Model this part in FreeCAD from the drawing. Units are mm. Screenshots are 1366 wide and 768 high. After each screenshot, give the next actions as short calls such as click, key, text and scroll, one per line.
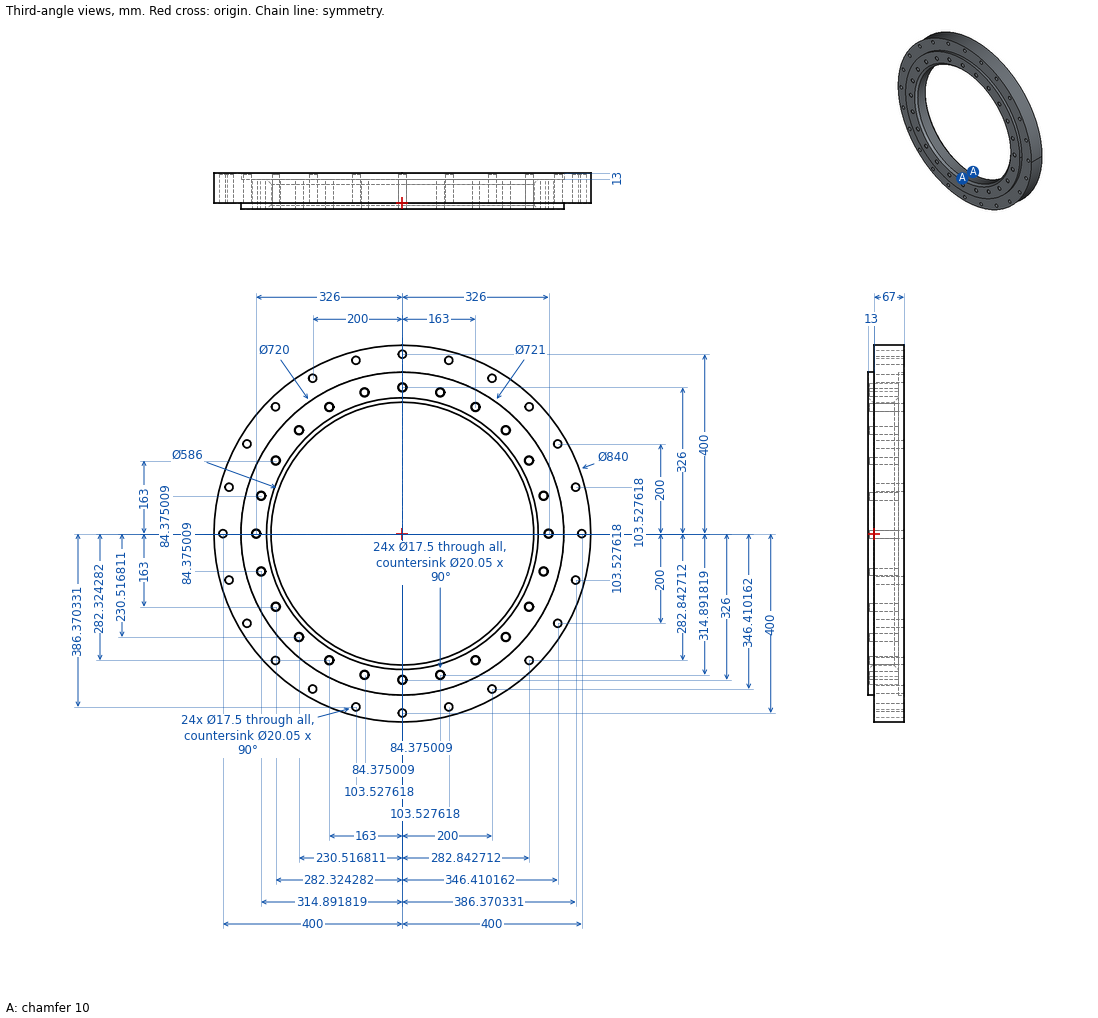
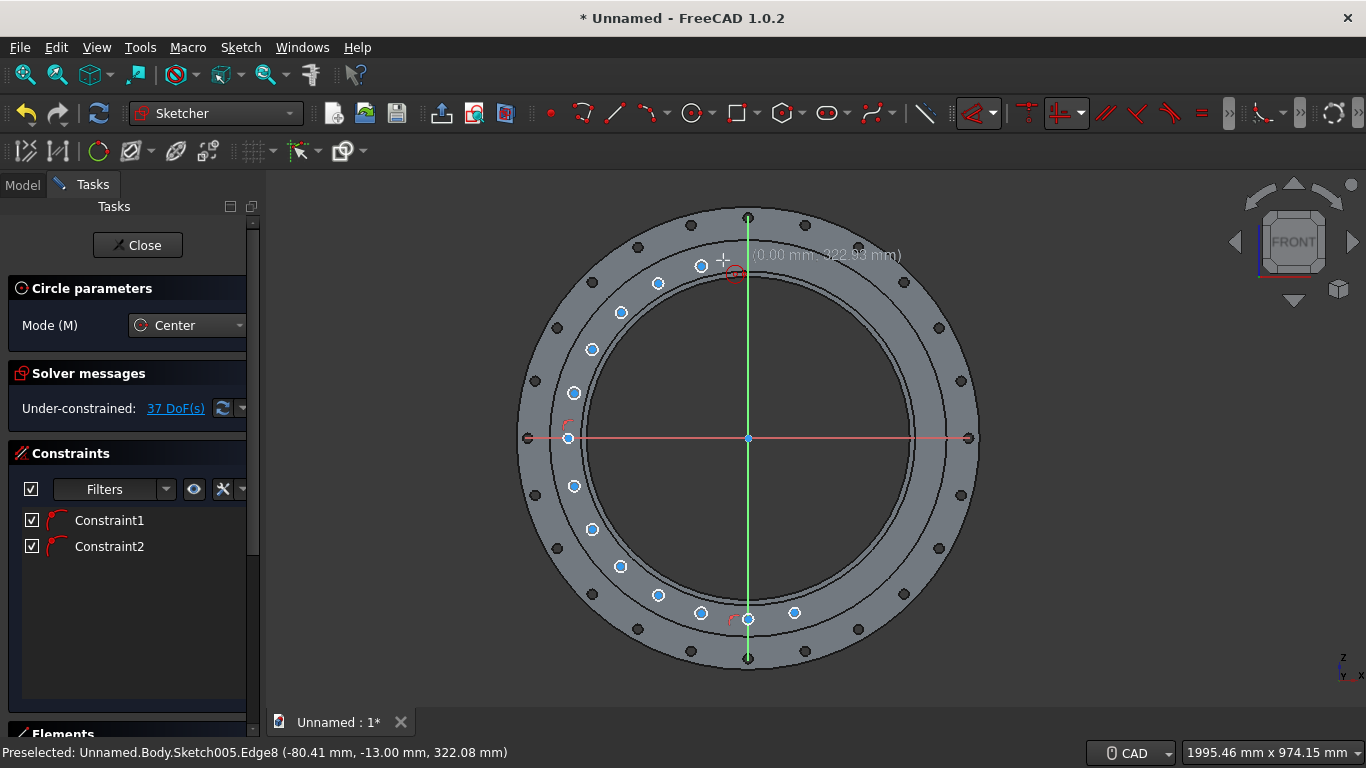
click(748, 259)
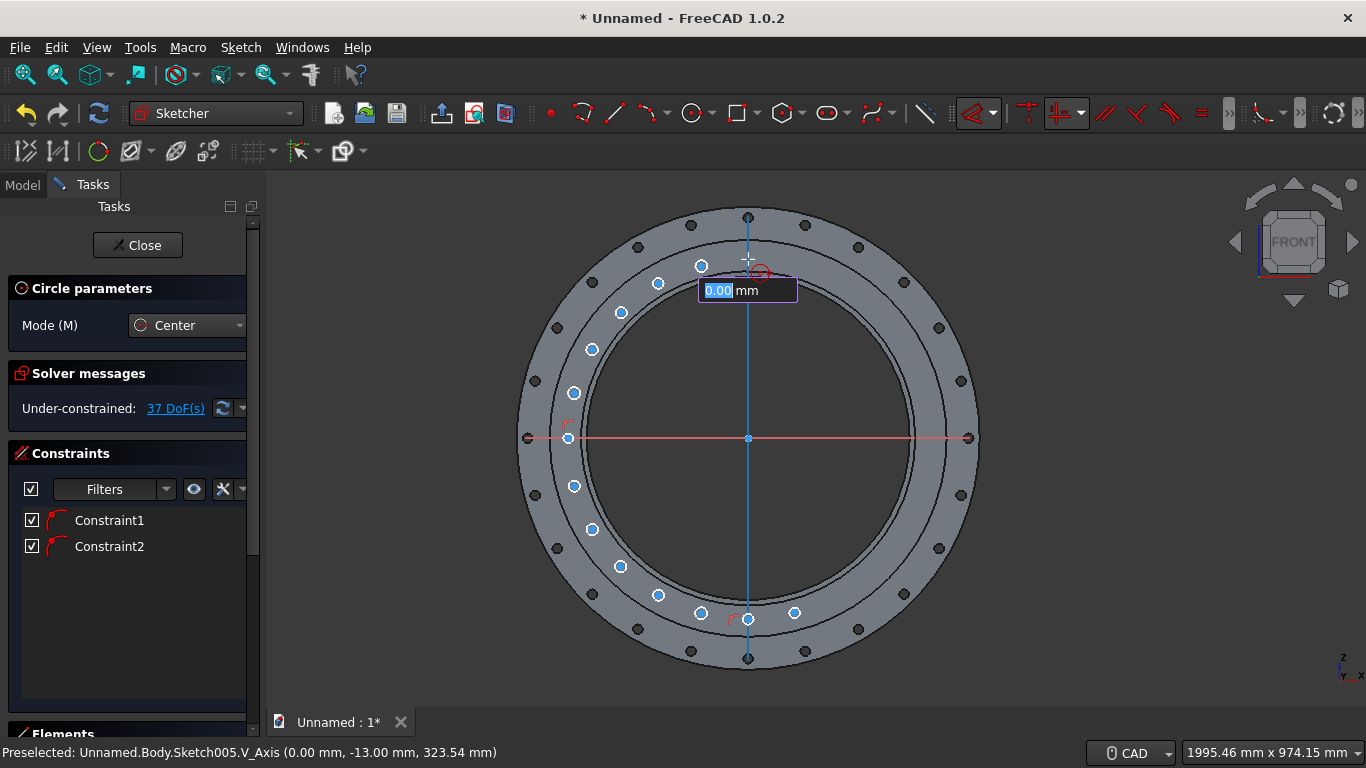
scroll(753, 257, up, 7)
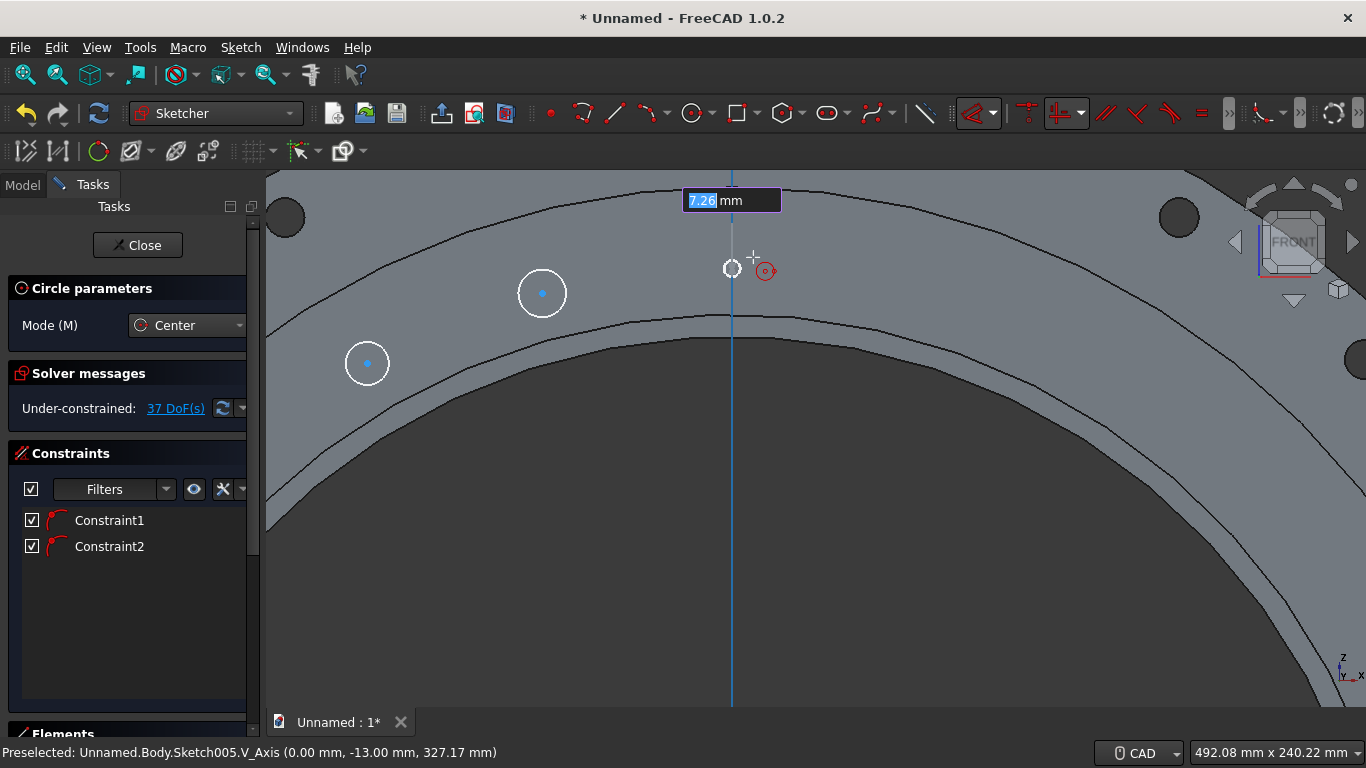
click(750, 256)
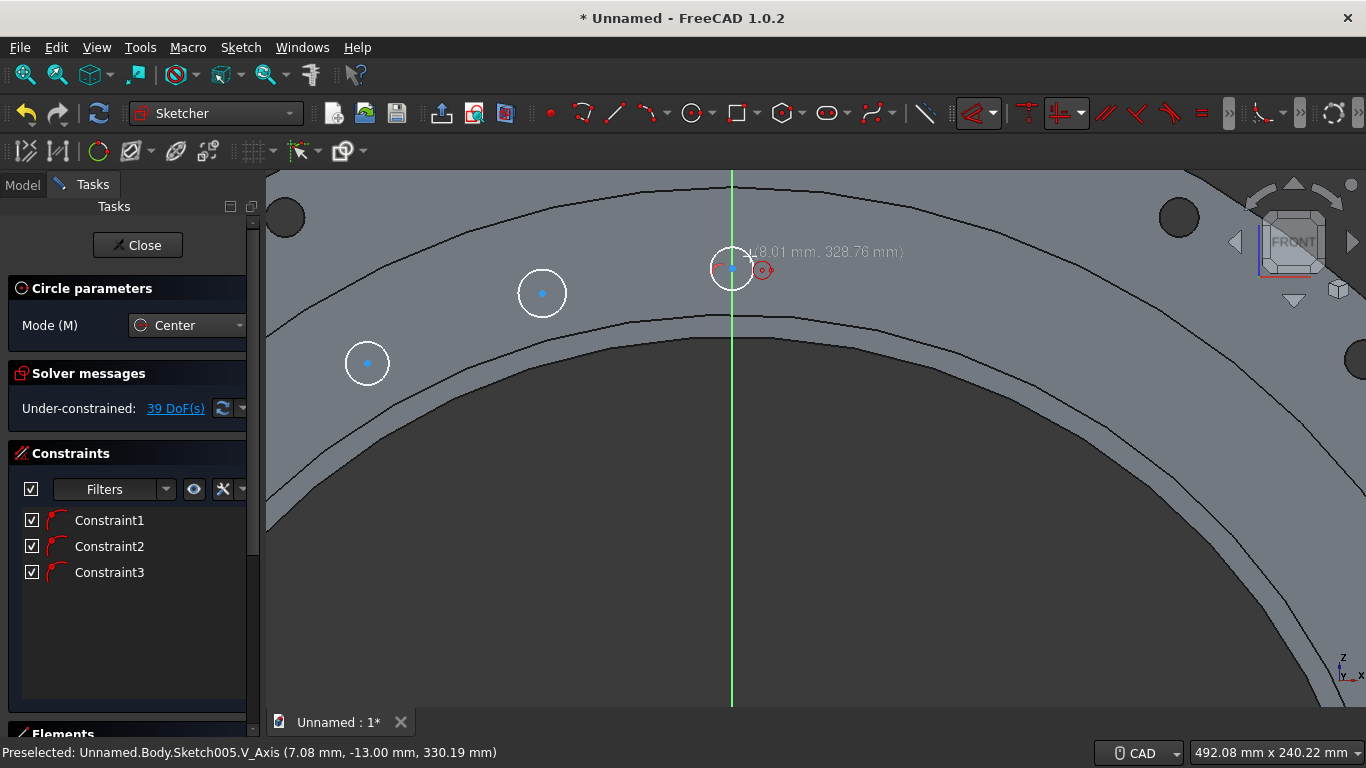
scroll(753, 257, down, 7)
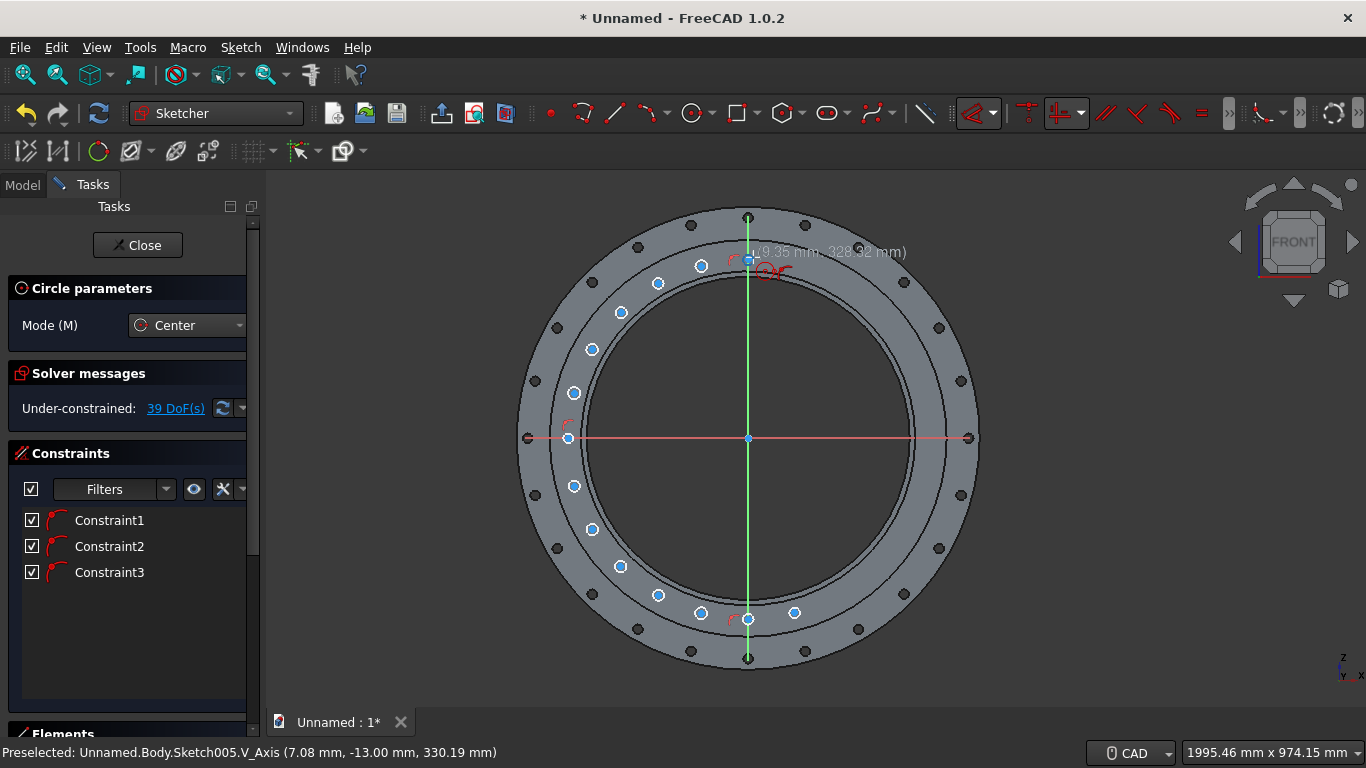
click(795, 265)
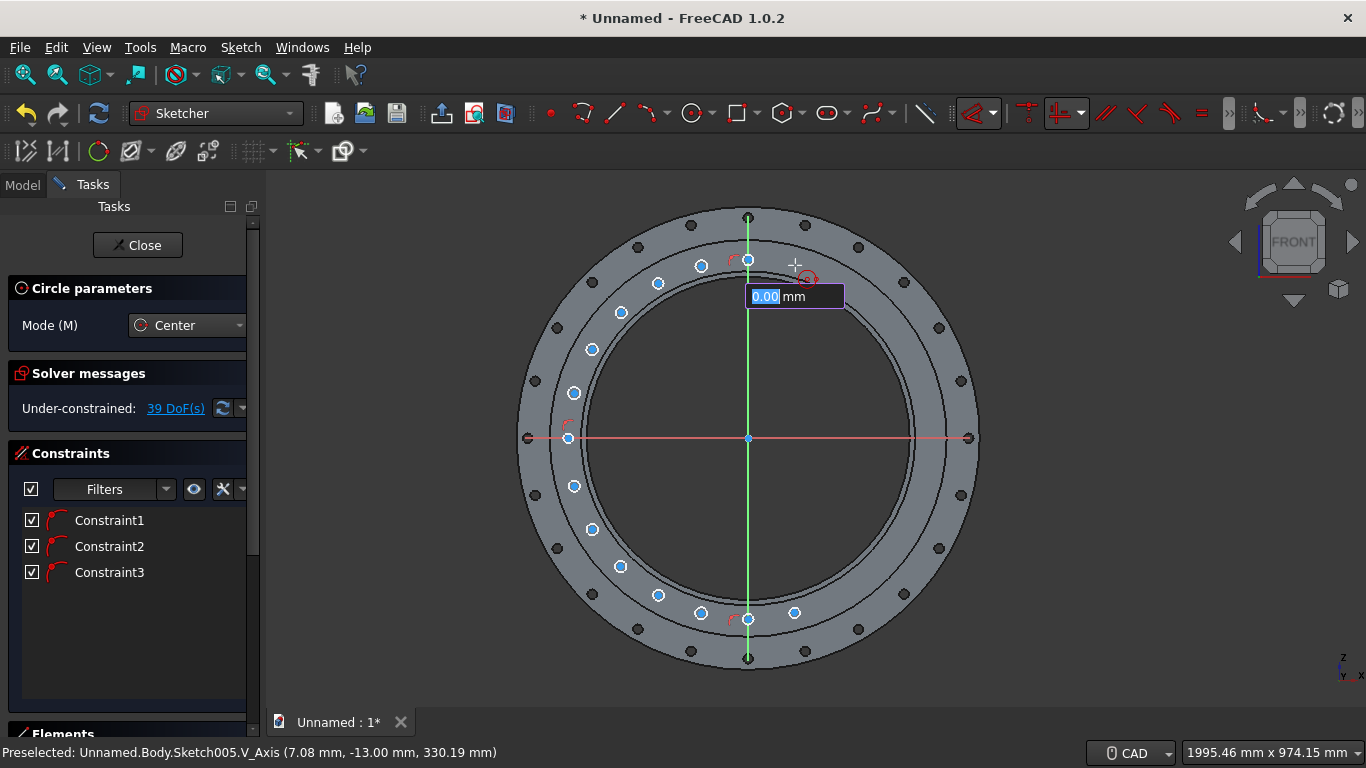
scroll(798, 261, up, 6)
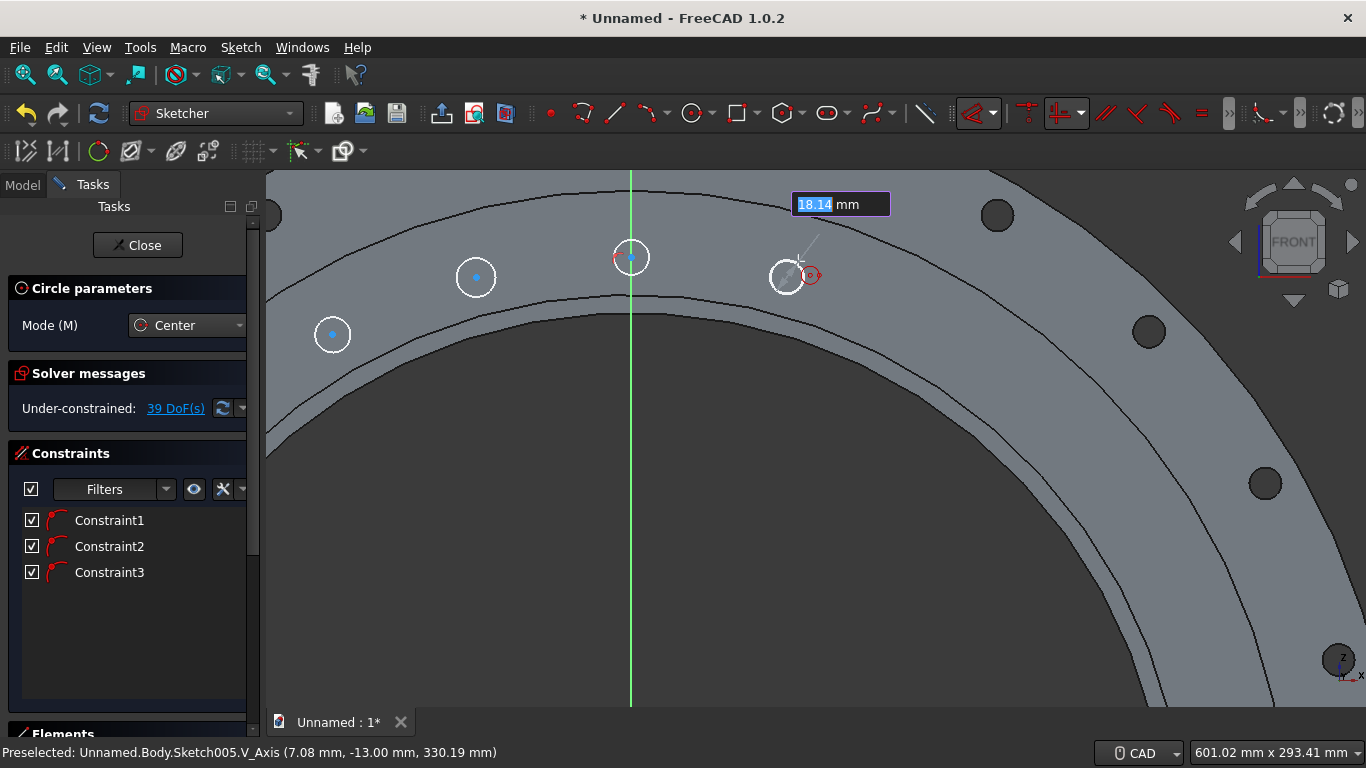
click(797, 262)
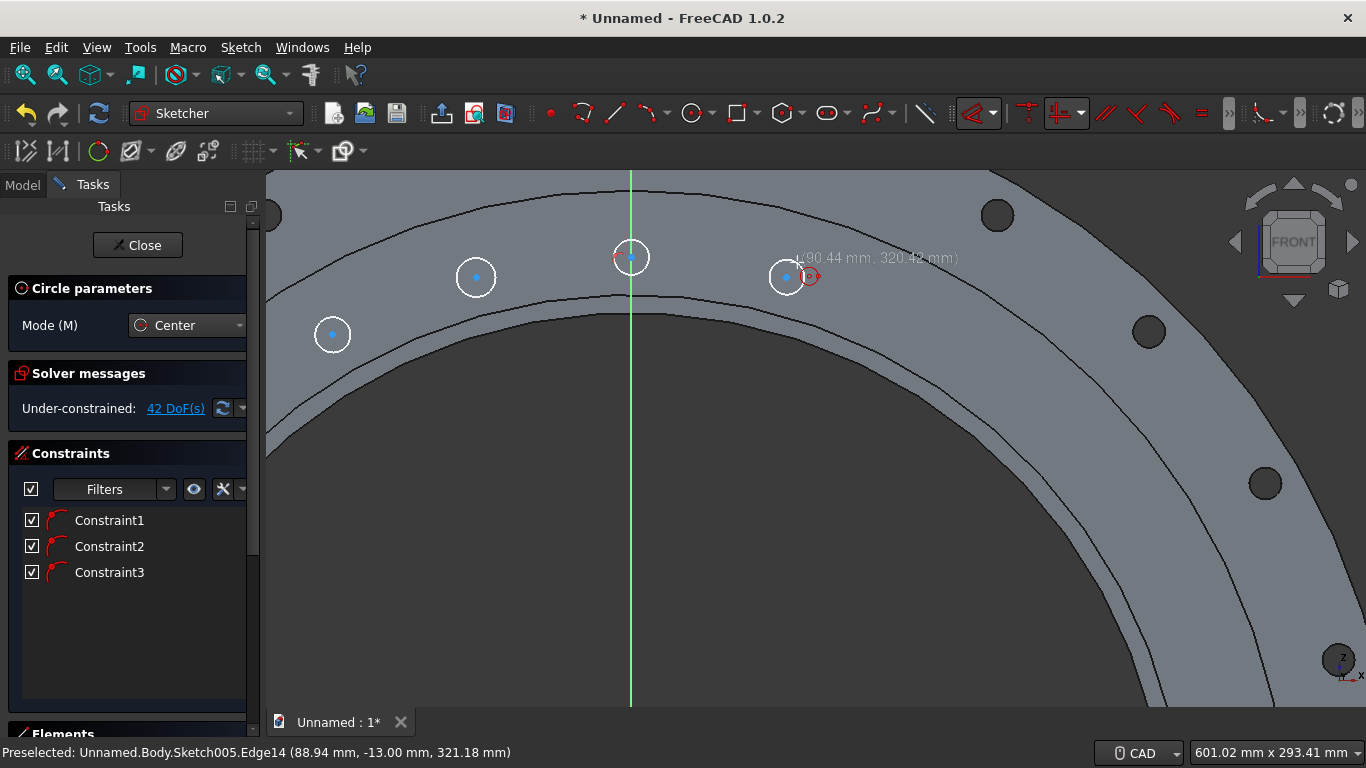
scroll(930, 333, up, 2)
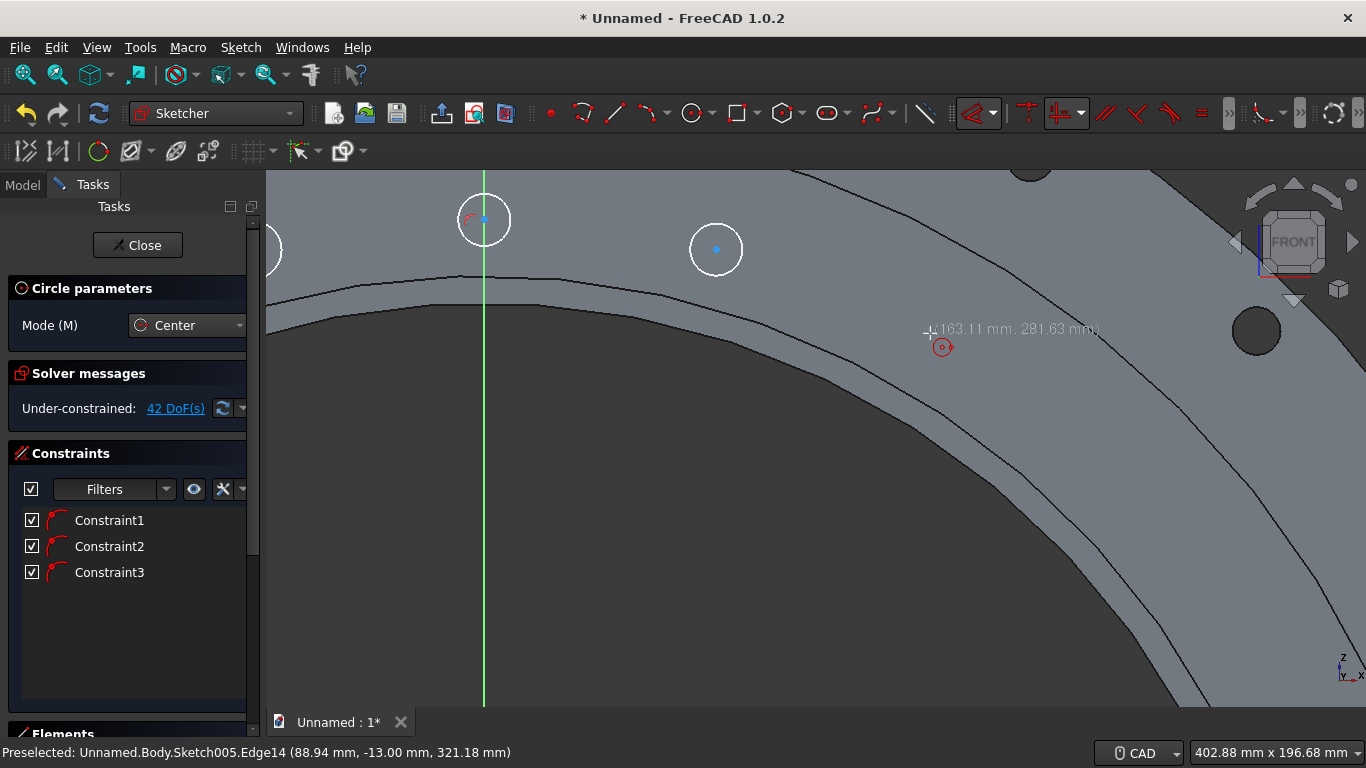
scroll(814, 270, down, 8)